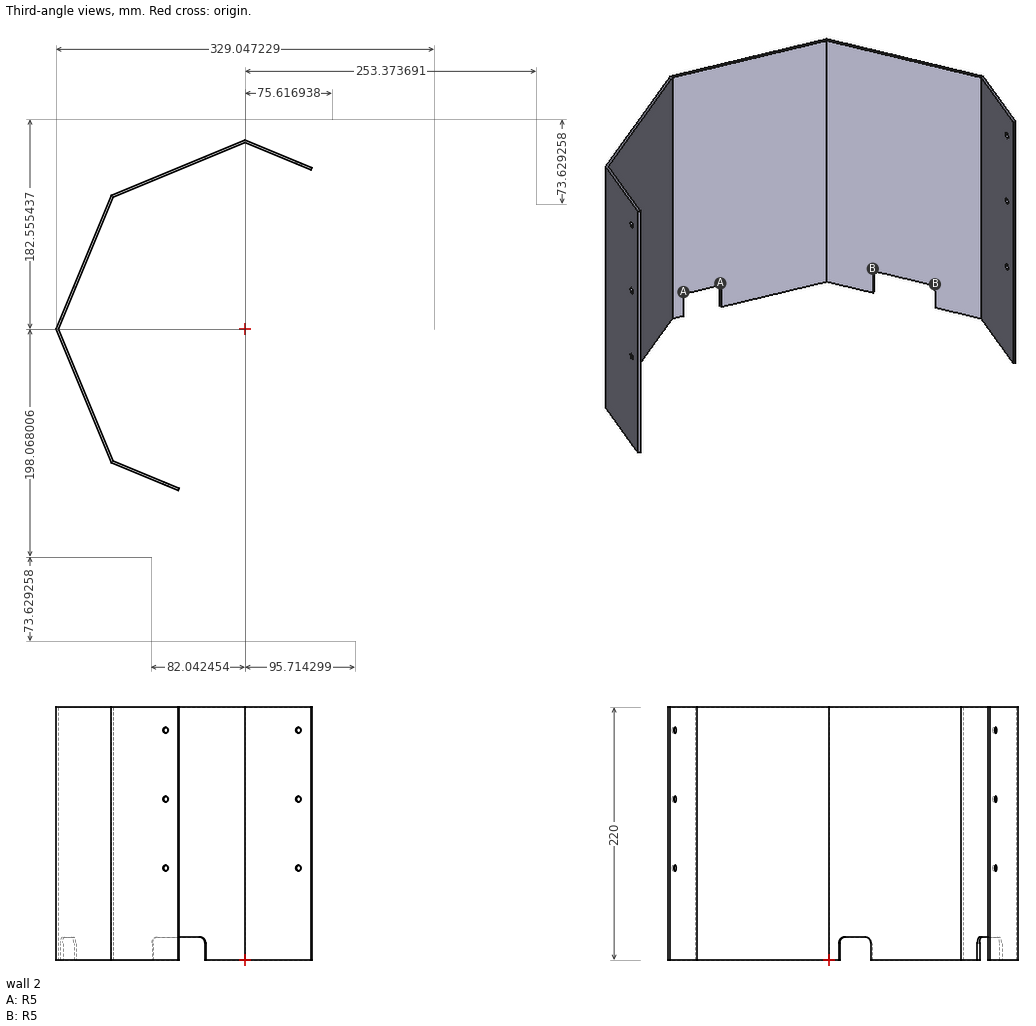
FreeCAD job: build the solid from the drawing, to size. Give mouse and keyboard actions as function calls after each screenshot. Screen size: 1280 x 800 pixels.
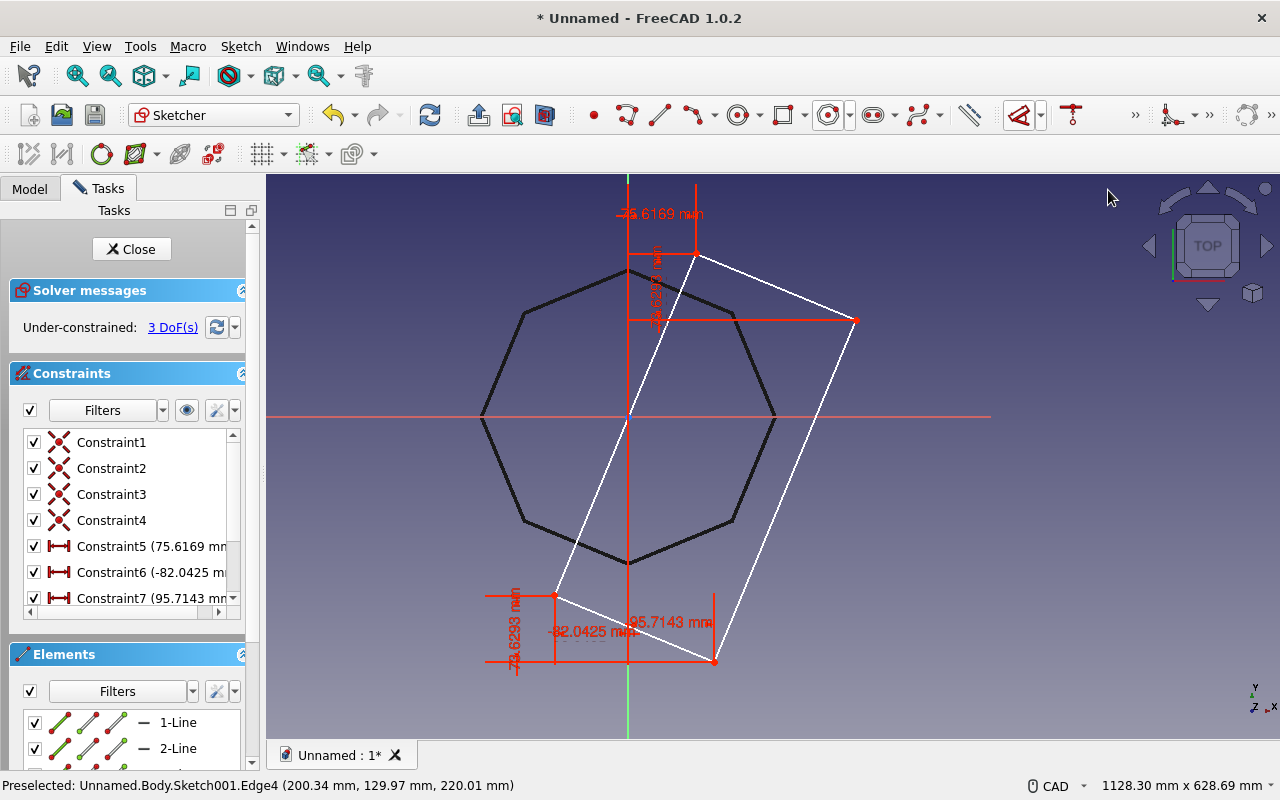
click(696, 254)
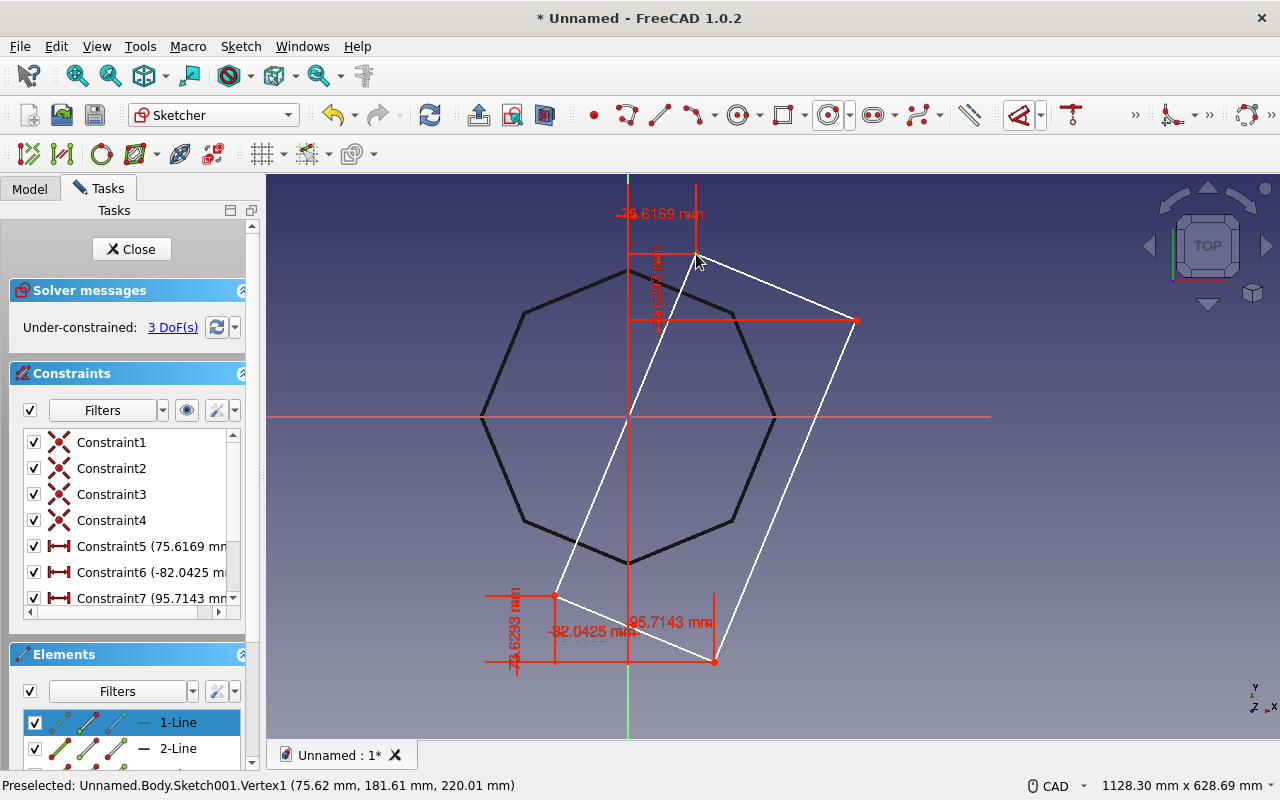
click(1040, 116)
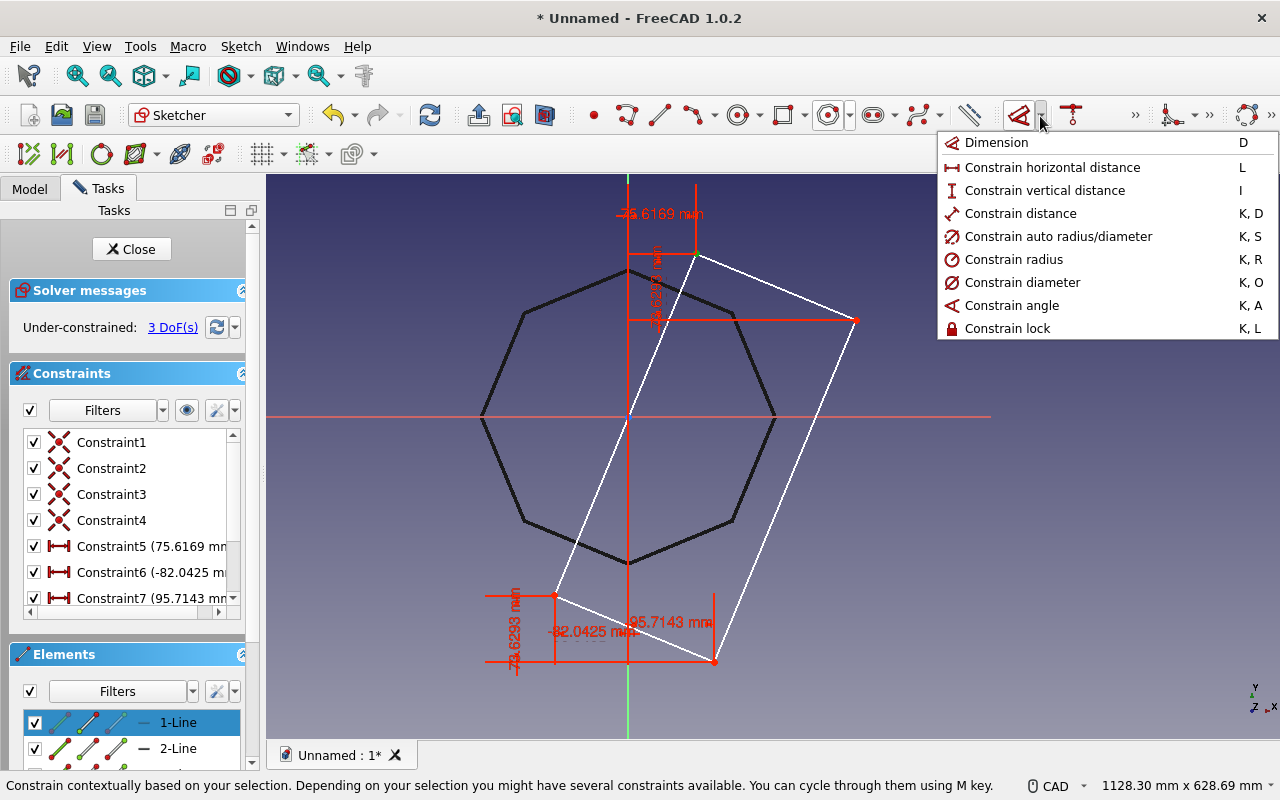
click(1108, 190)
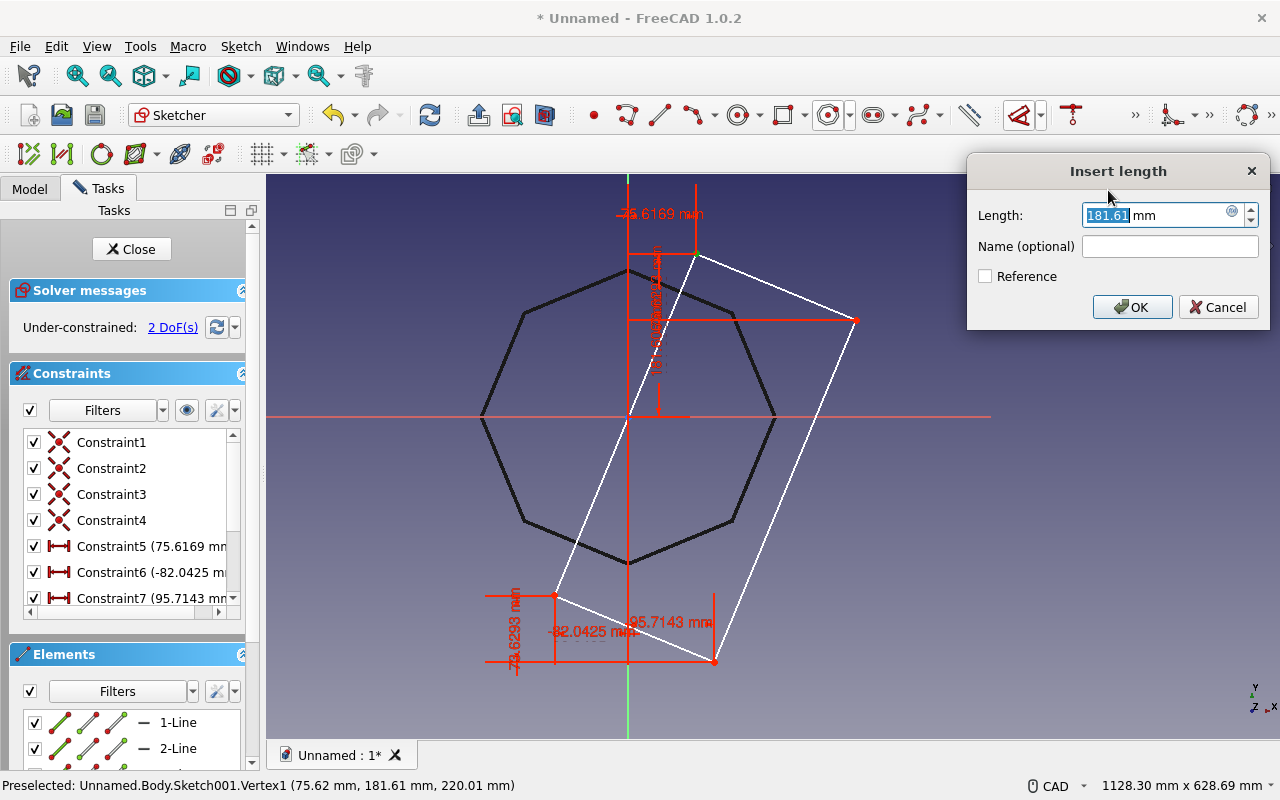
text(182.555437)
key(Return)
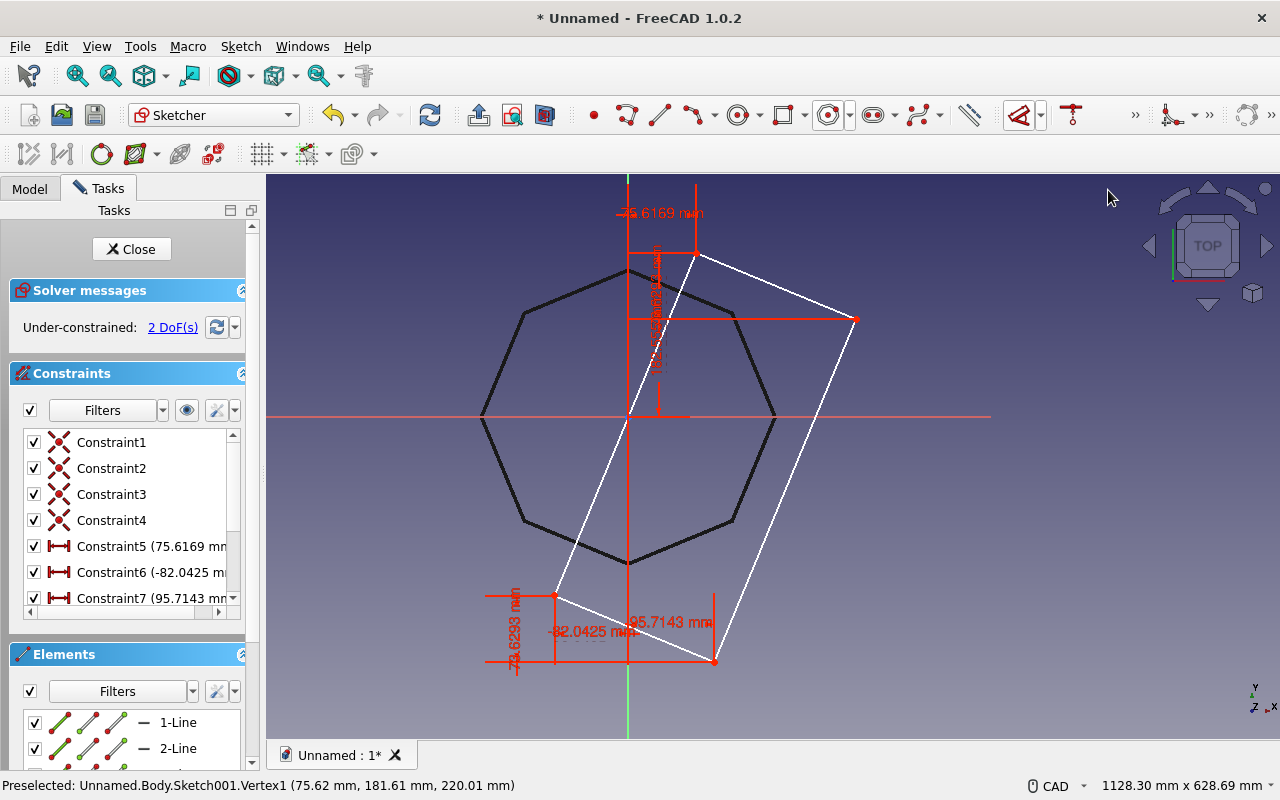
click(555, 596)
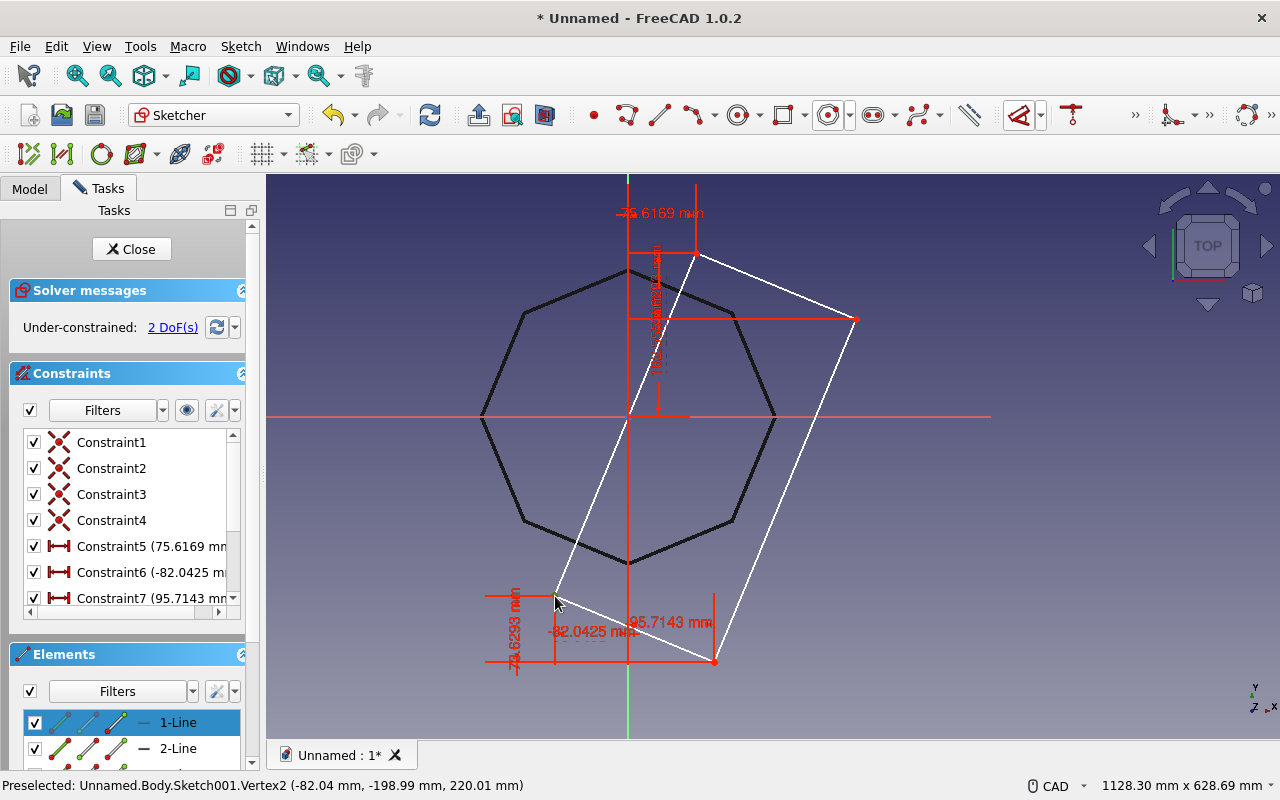
click(1040, 116)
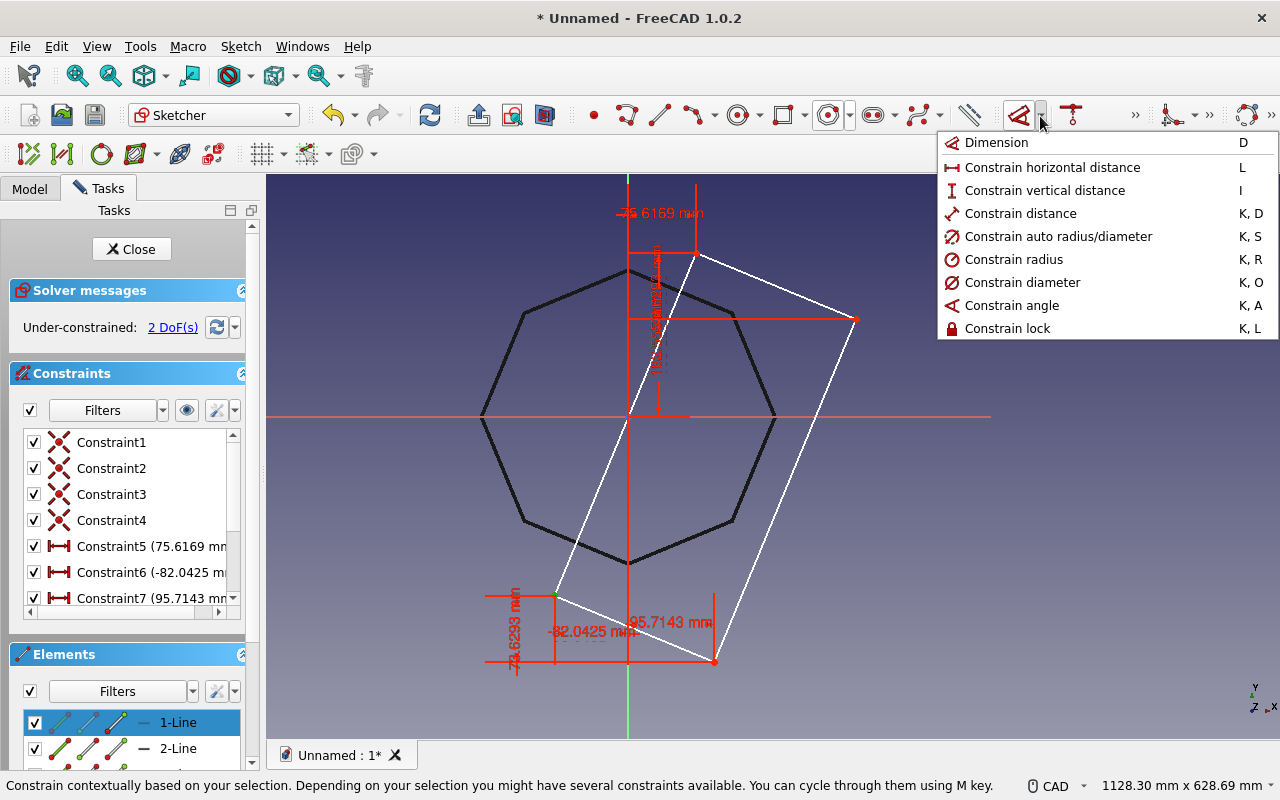
click(1108, 190)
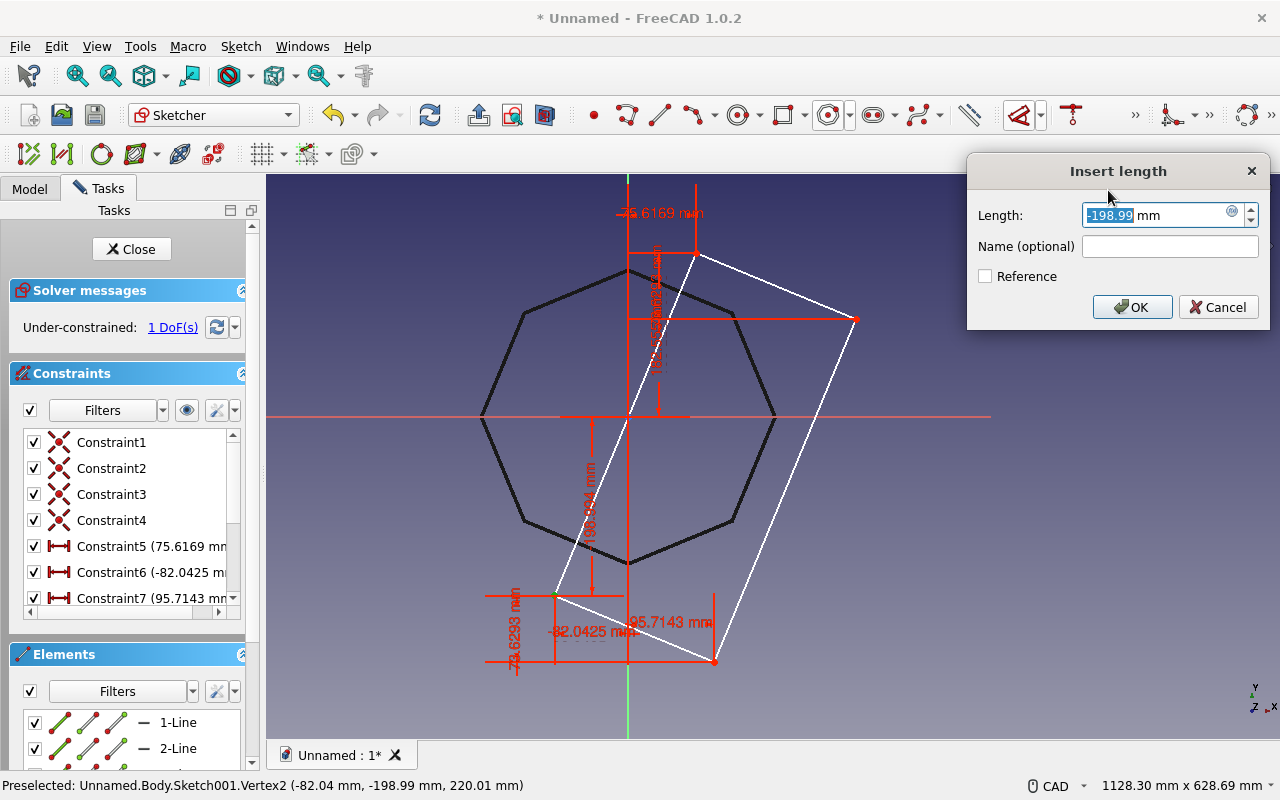
text(-198.068006)
key(Return)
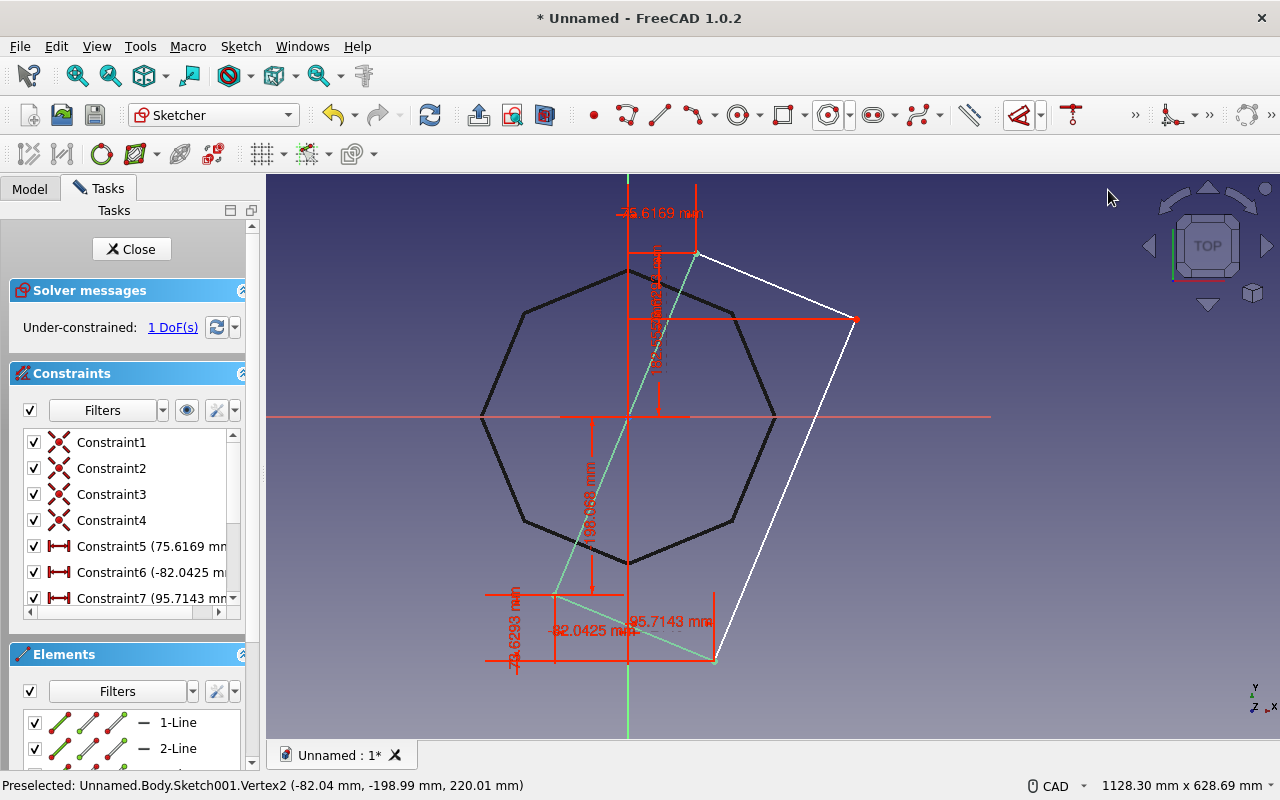
click(856, 319)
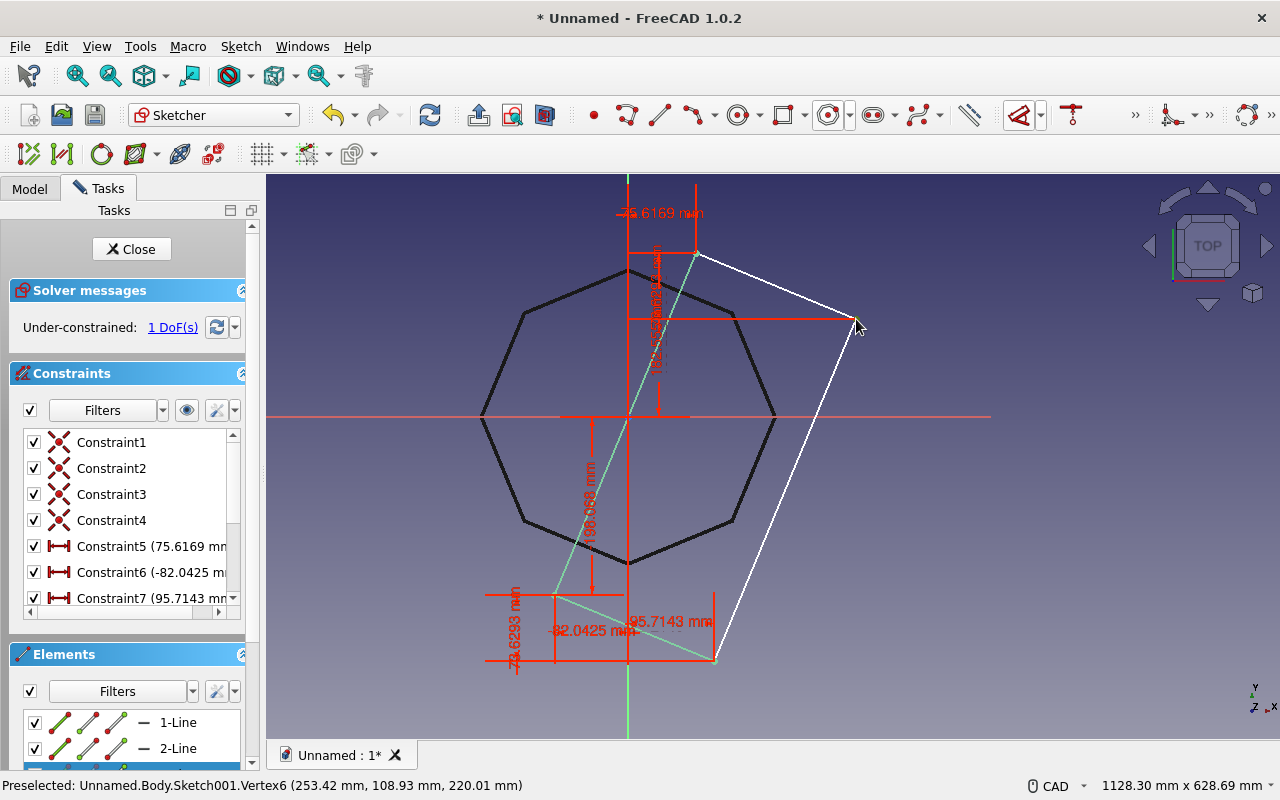
click(1040, 116)